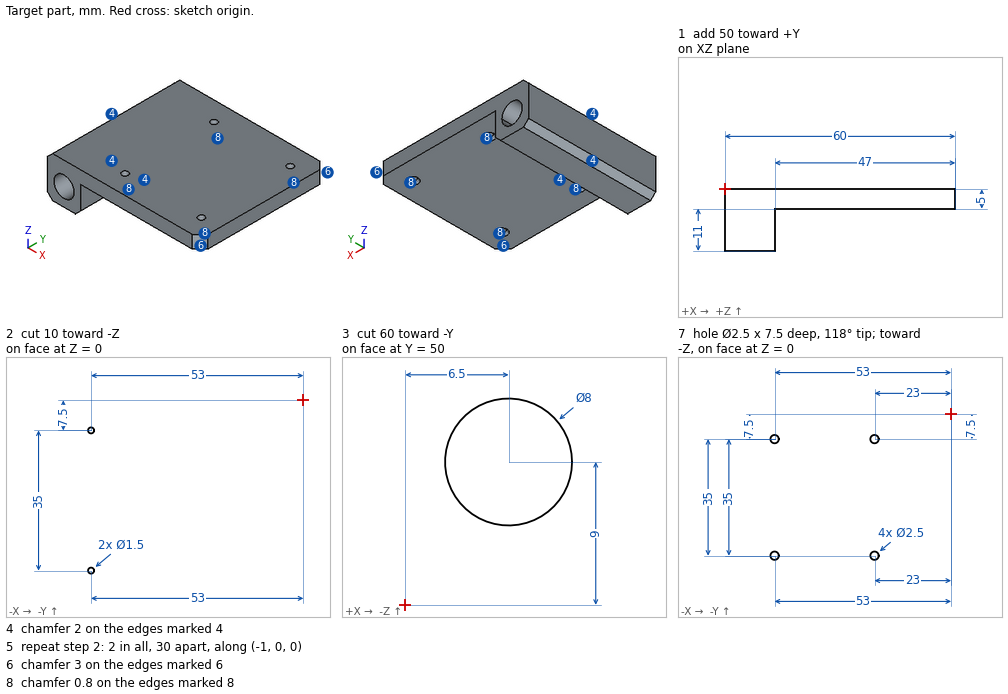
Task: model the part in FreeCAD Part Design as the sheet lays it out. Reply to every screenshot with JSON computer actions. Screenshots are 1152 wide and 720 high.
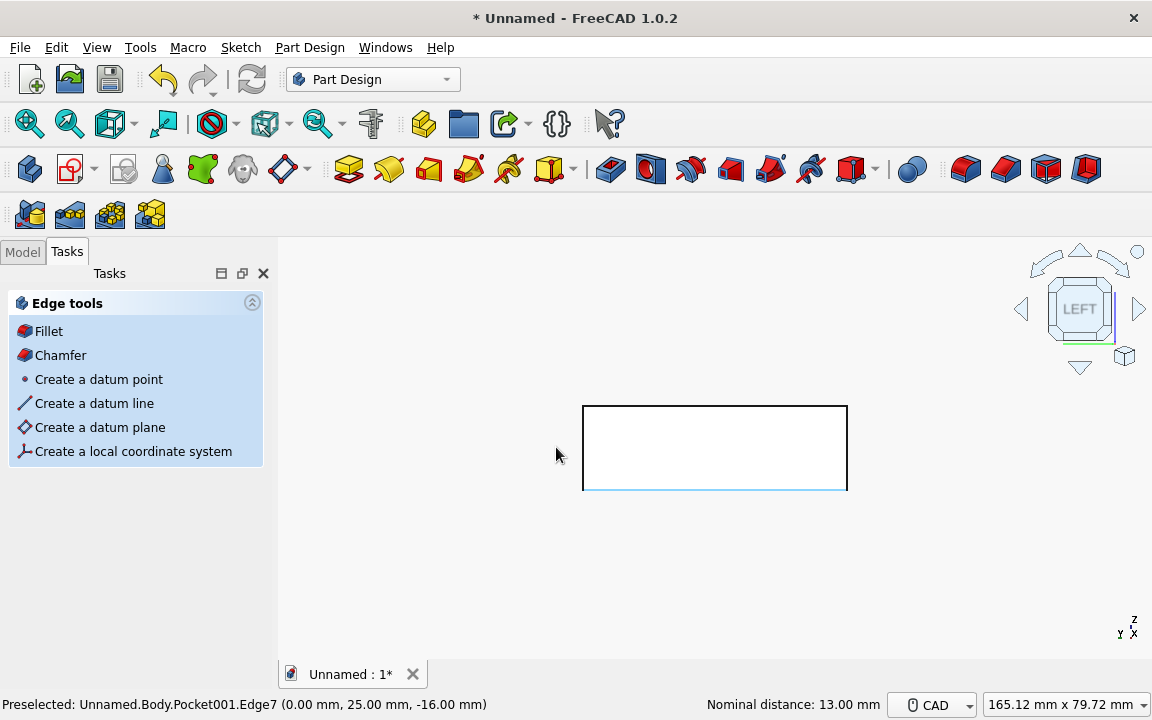
{"action": "left_click", "coordinate": [30, 124]}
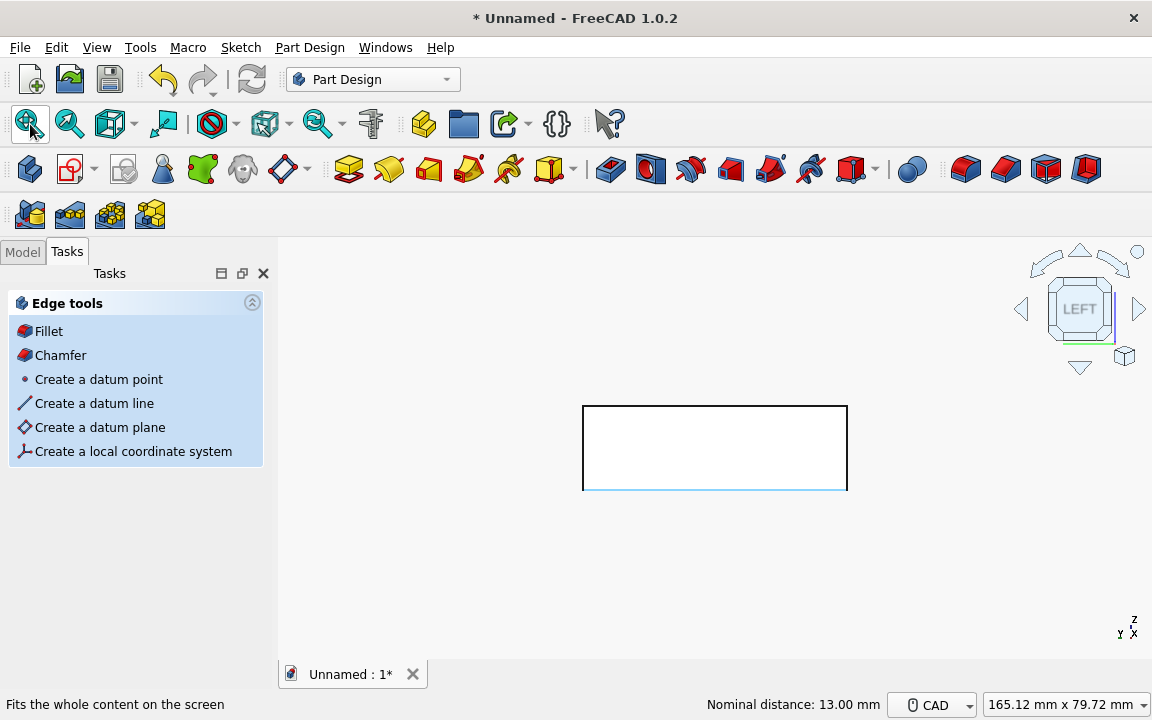
{"action": "key", "text": "v 3"}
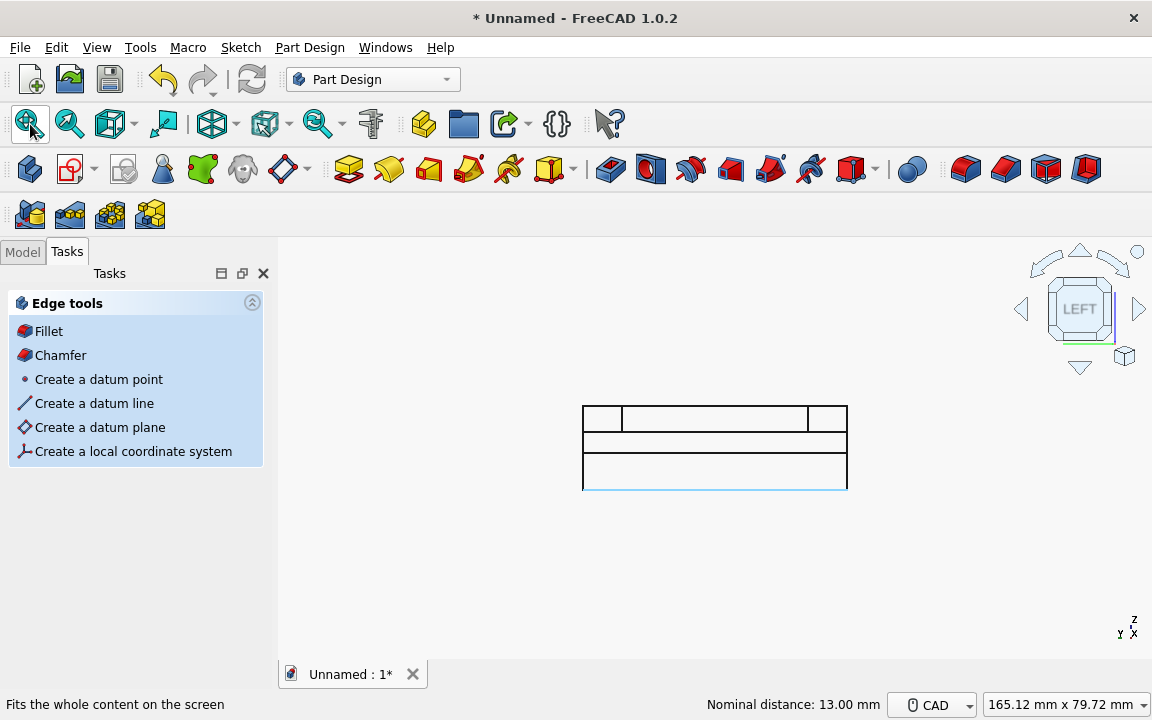
{"action": "key", "text": "0"}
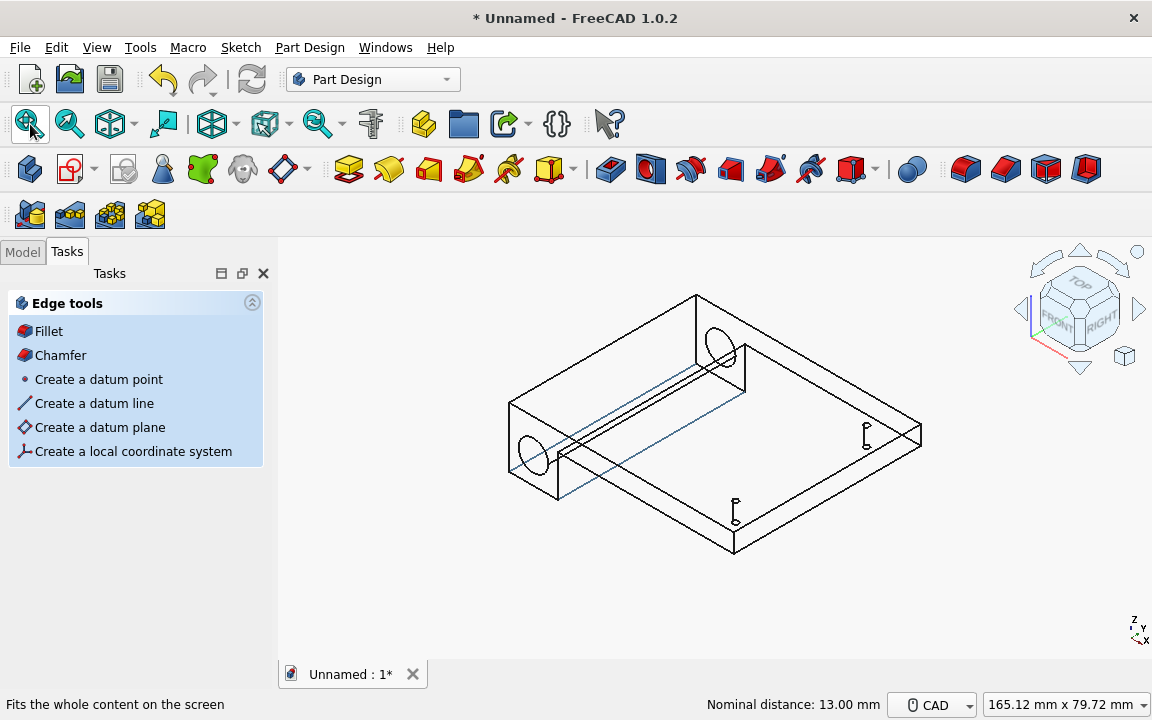
{"action": "left_click", "coordinate": [603, 348], "text": "ctrl"}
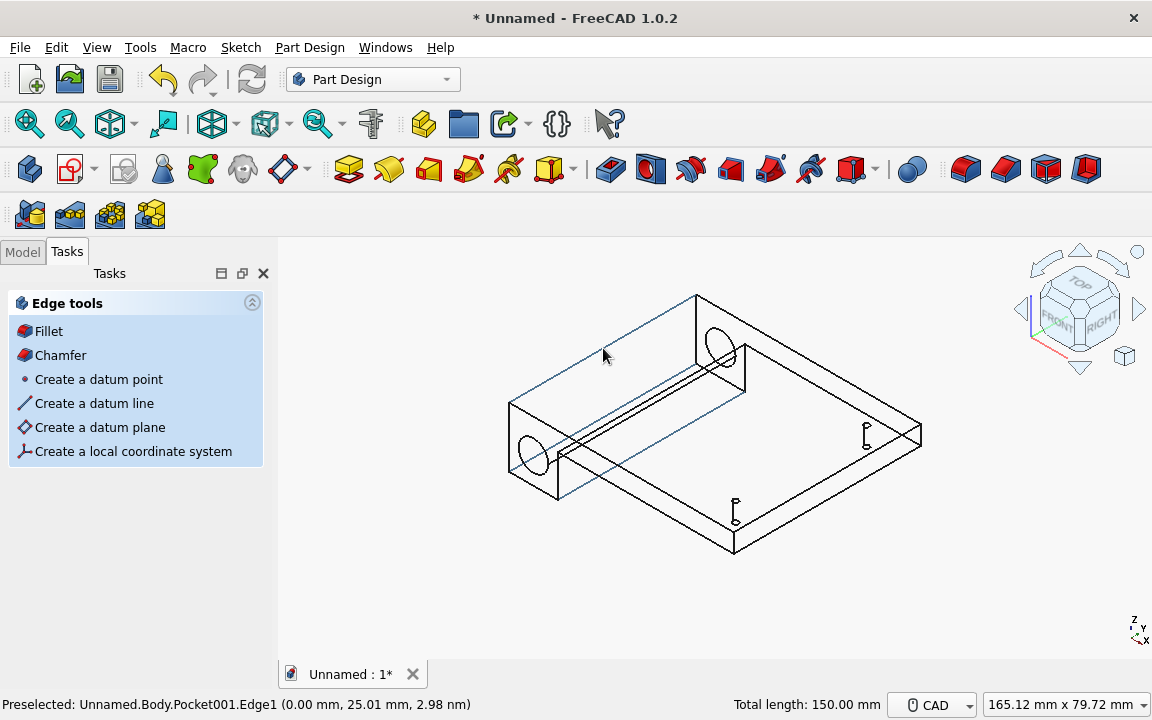
{"action": "key", "text": "v 1"}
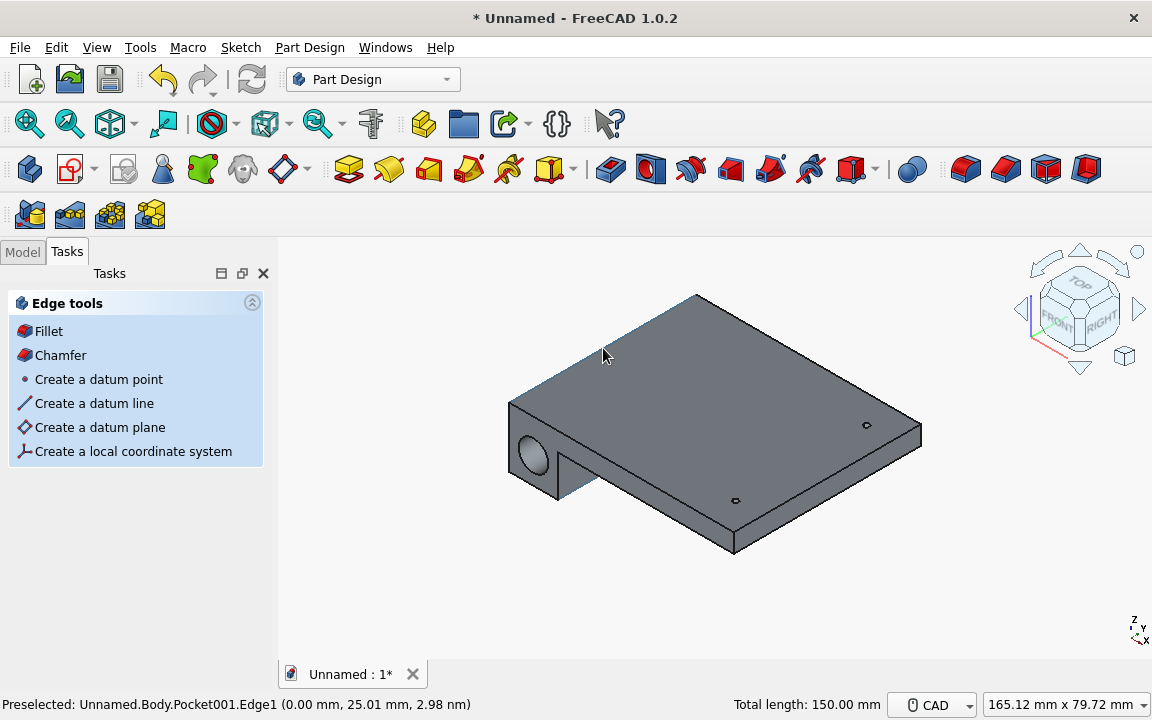
{"action": "left_click", "coordinate": [1006, 170]}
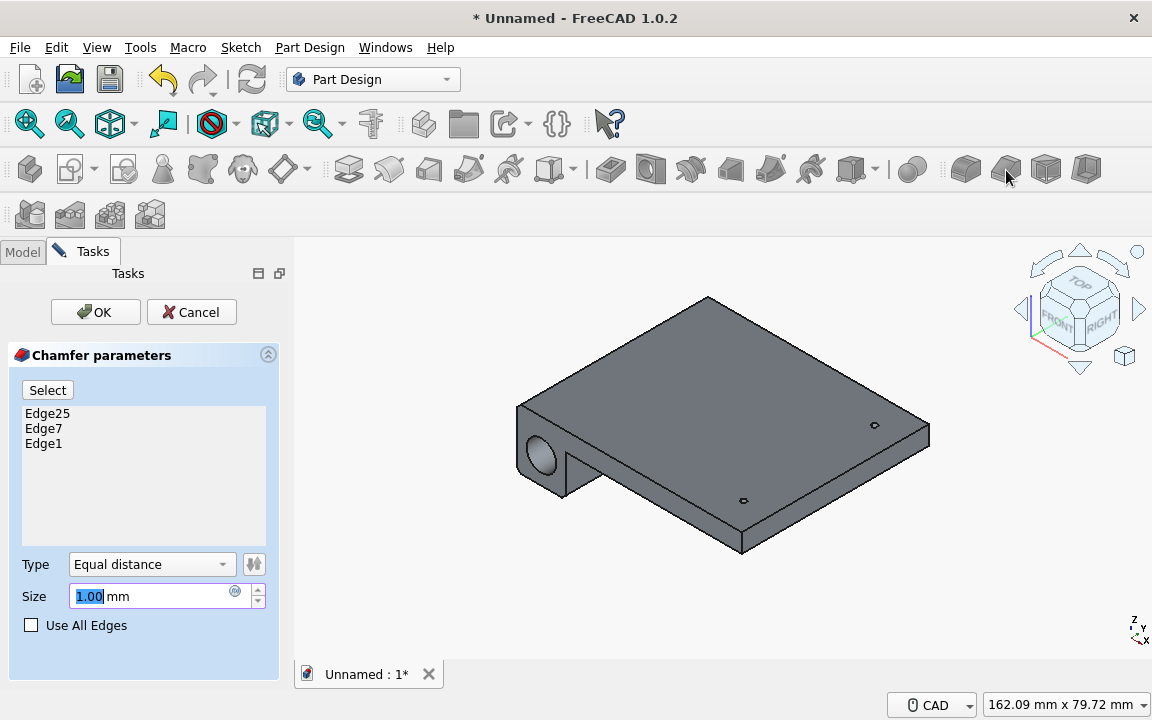
{"action": "type", "text": "2"}
{"action": "key", "text": "Tab"}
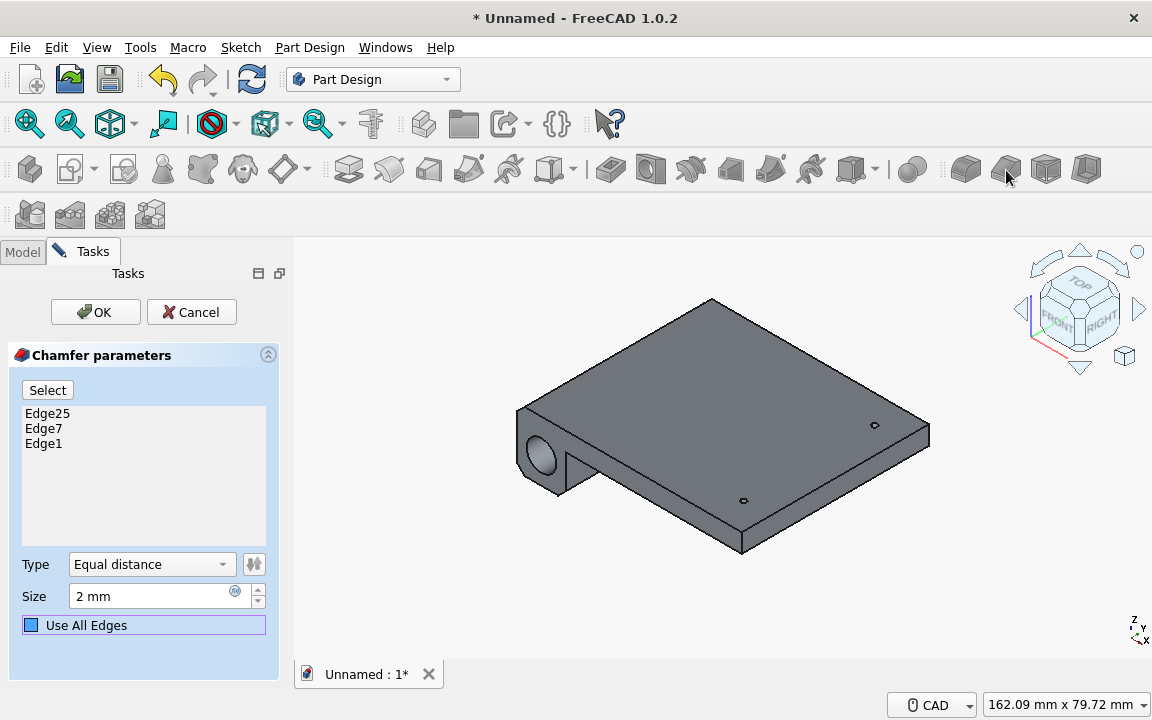
{"action": "left_click", "coordinate": [96, 312]}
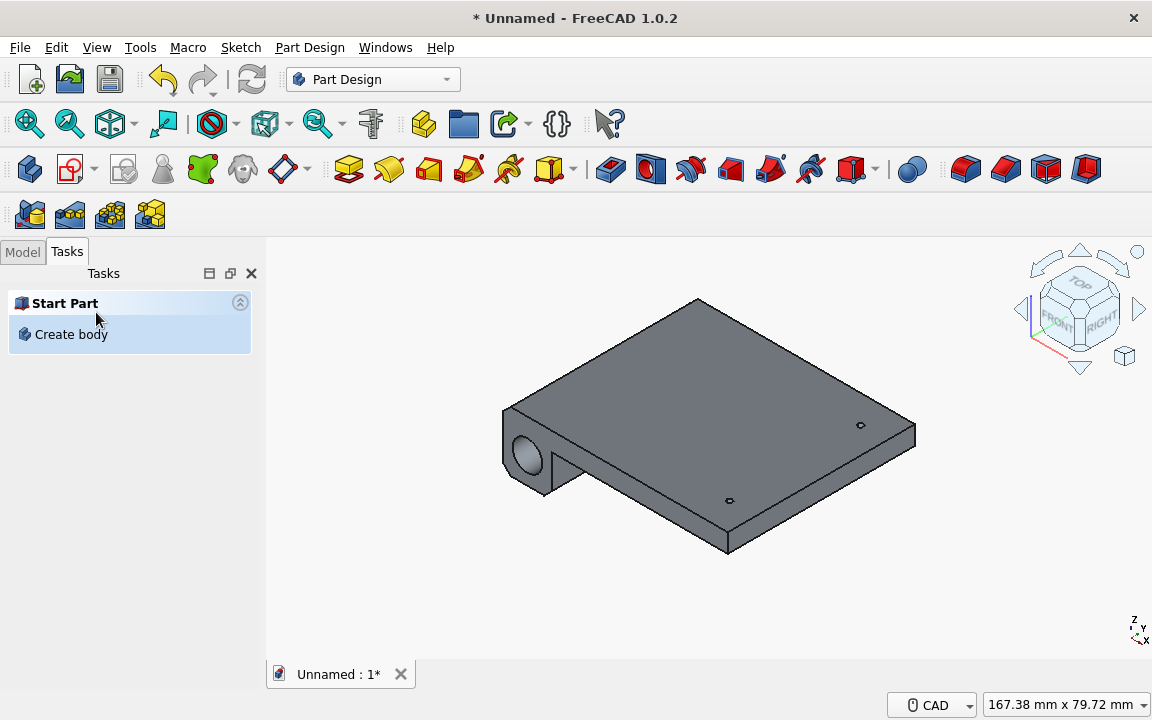
{"action": "left_click", "coordinate": [23, 251]}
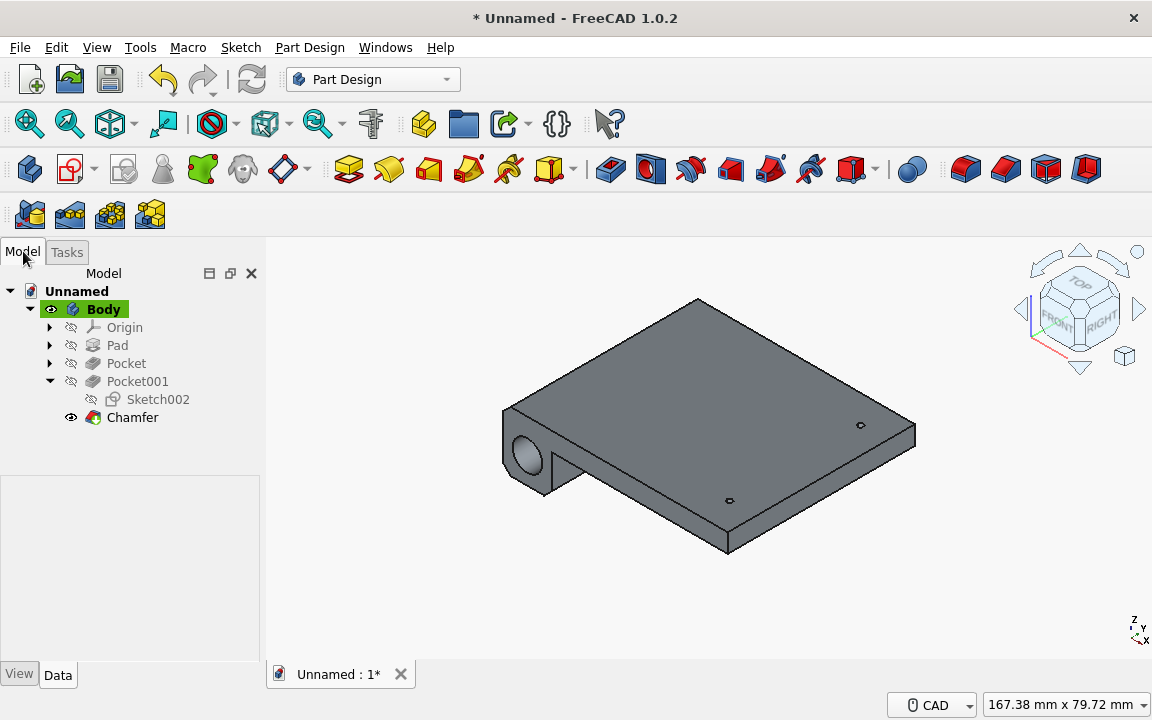
{"action": "left_click", "coordinate": [116, 363]}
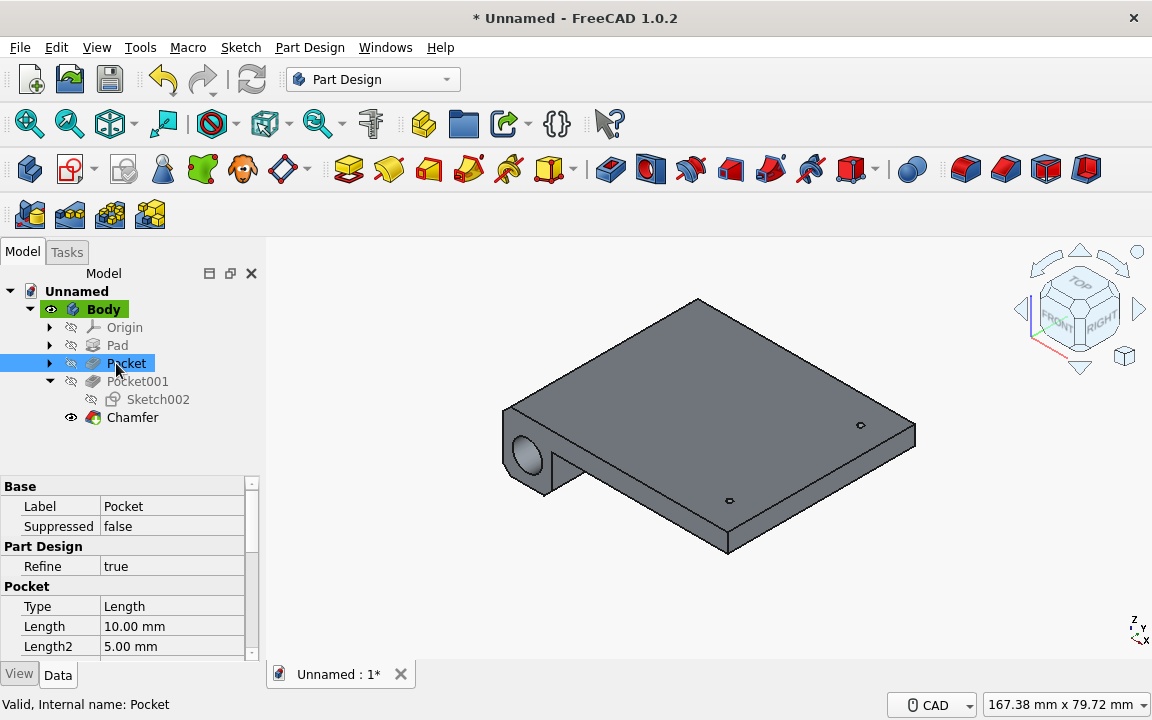
{"action": "left_click", "coordinate": [70, 214]}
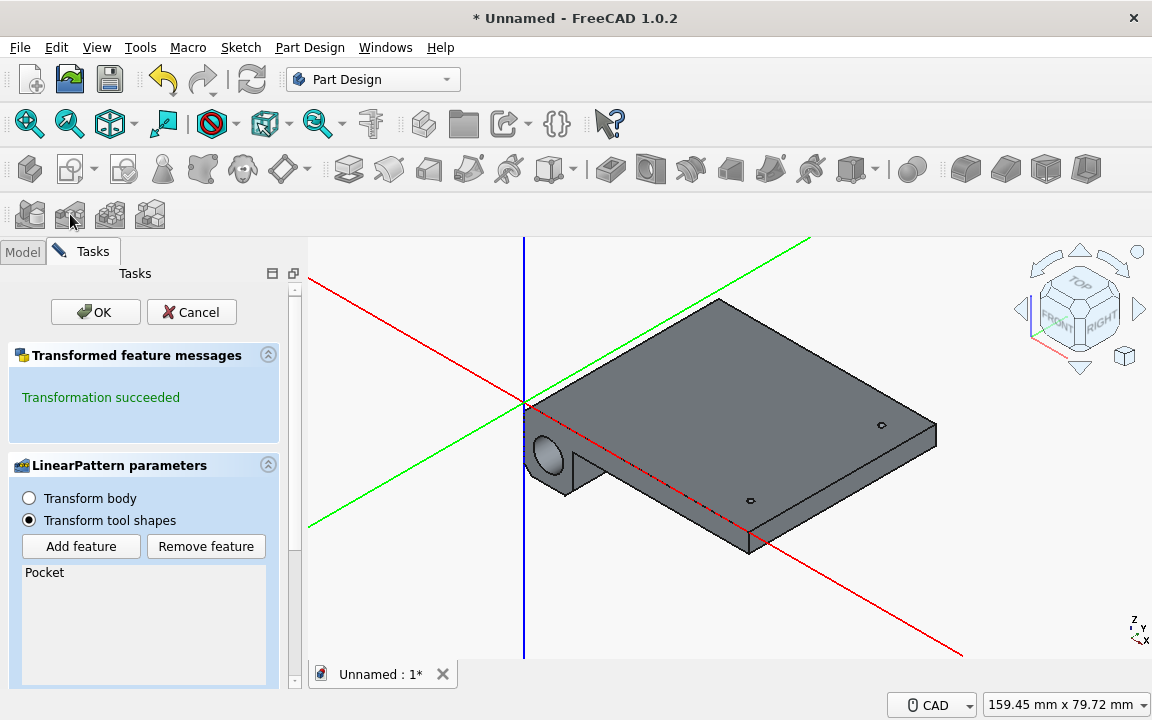
{"action": "scroll", "coordinate": [295, 486], "scroll_direction": "down", "scroll_amount": 2}